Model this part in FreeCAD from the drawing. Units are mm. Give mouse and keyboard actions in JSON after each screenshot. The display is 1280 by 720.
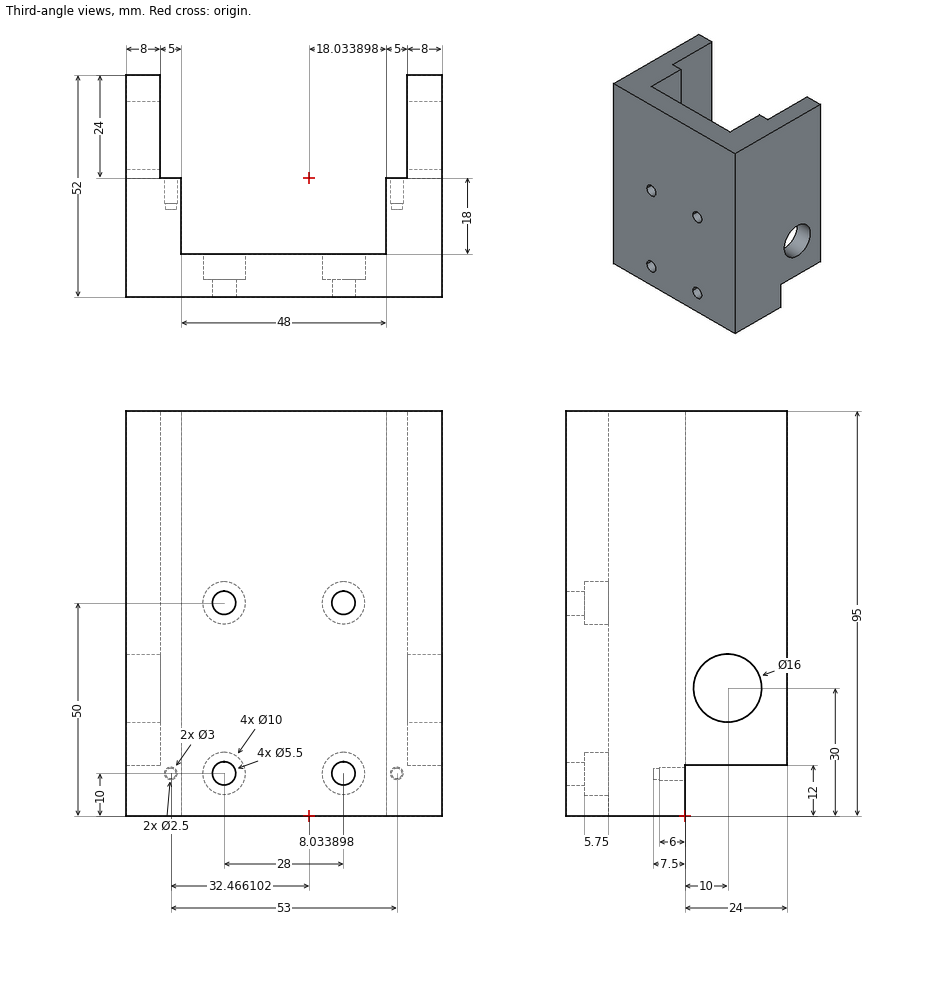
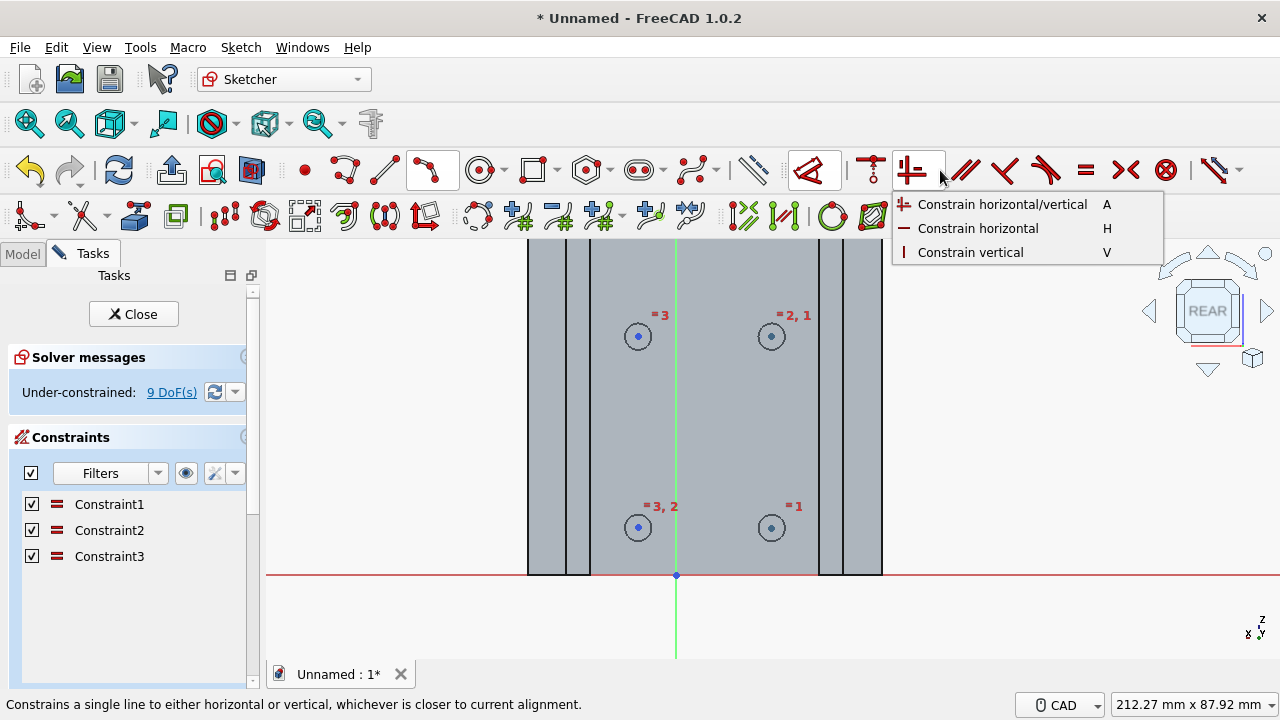
{"action": "left_click", "coordinate": [1028, 252]}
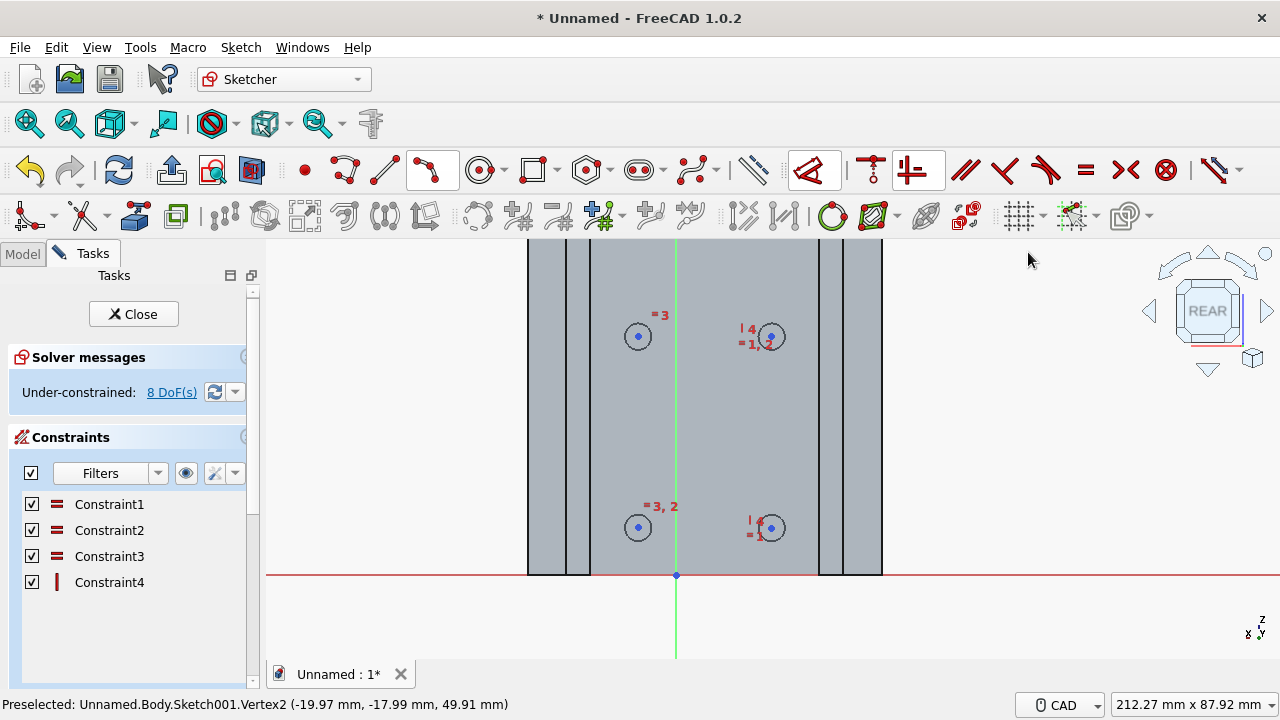
{"action": "left_click", "coordinate": [772, 528]}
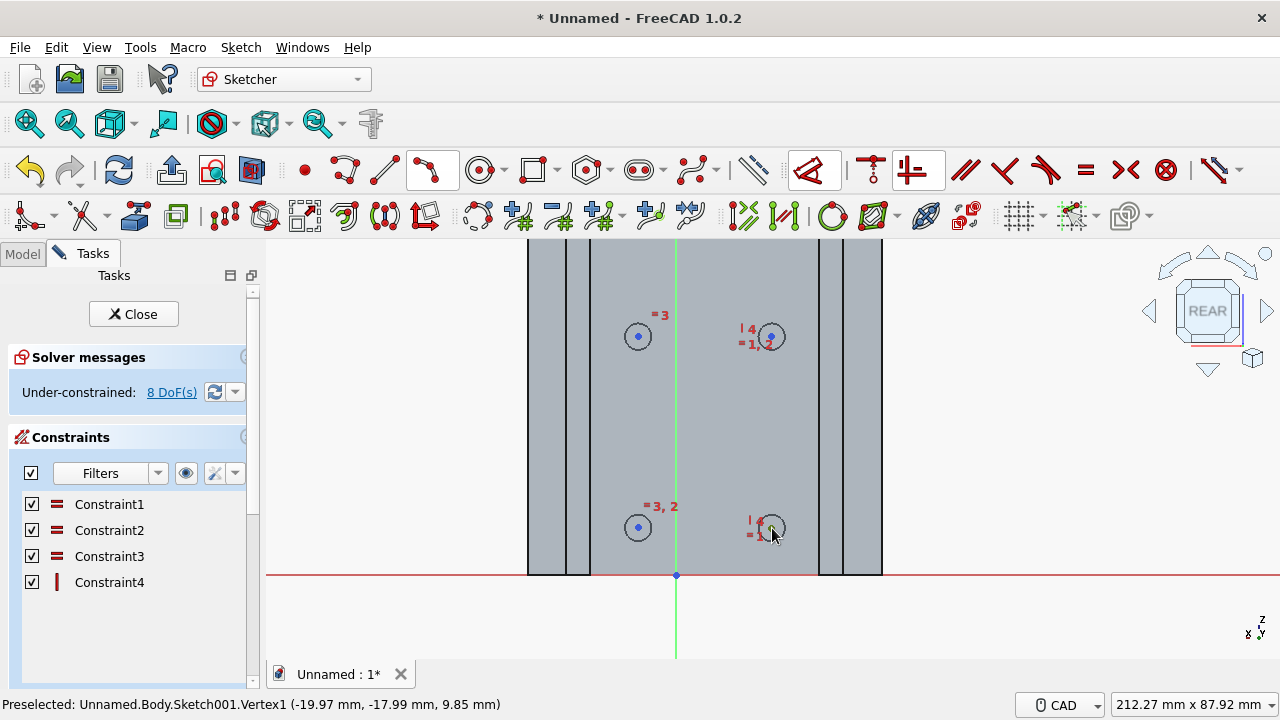
{"action": "left_click", "coordinate": [638, 528]}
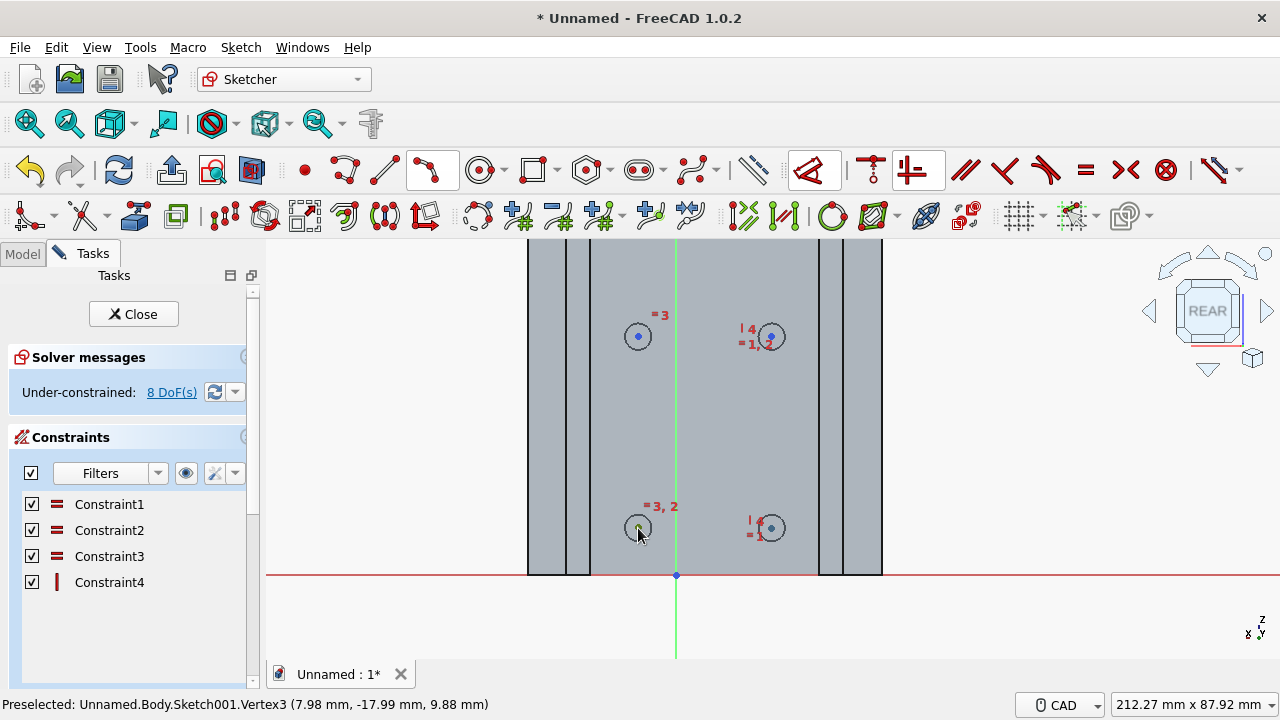
{"action": "key", "text": "h"}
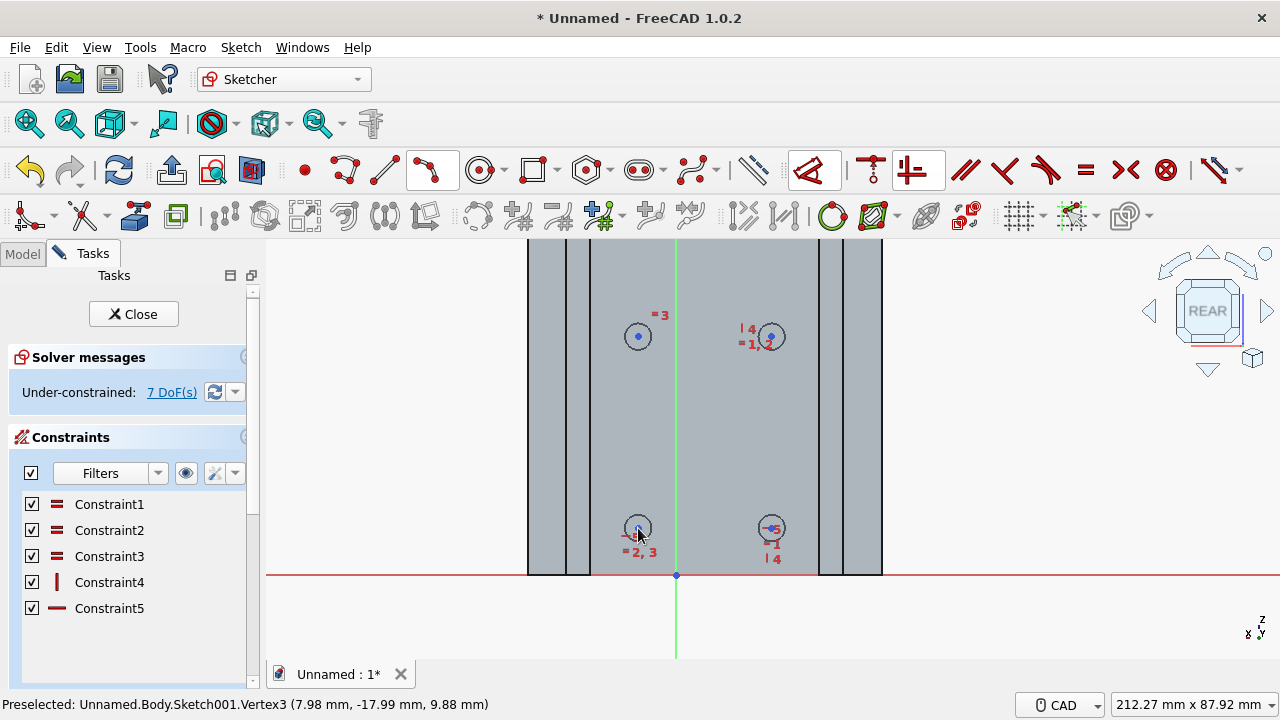
{"action": "left_click", "coordinate": [638, 528]}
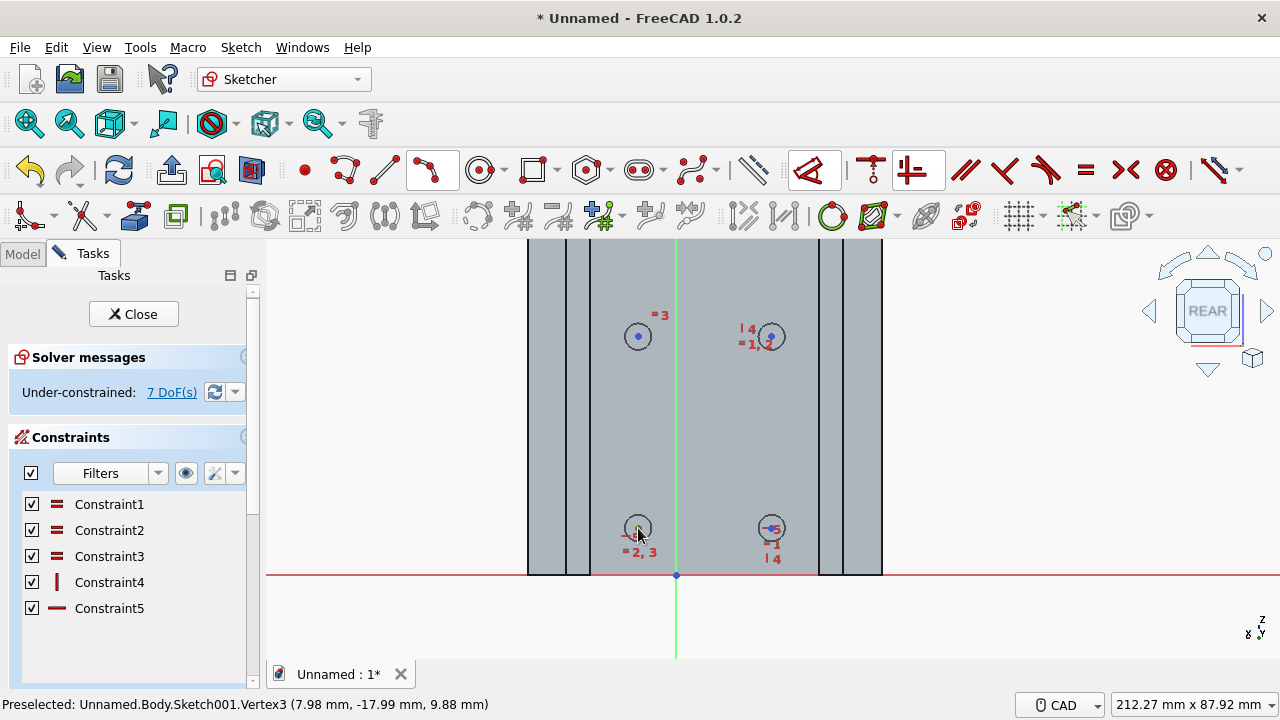
{"action": "left_click", "coordinate": [638, 337]}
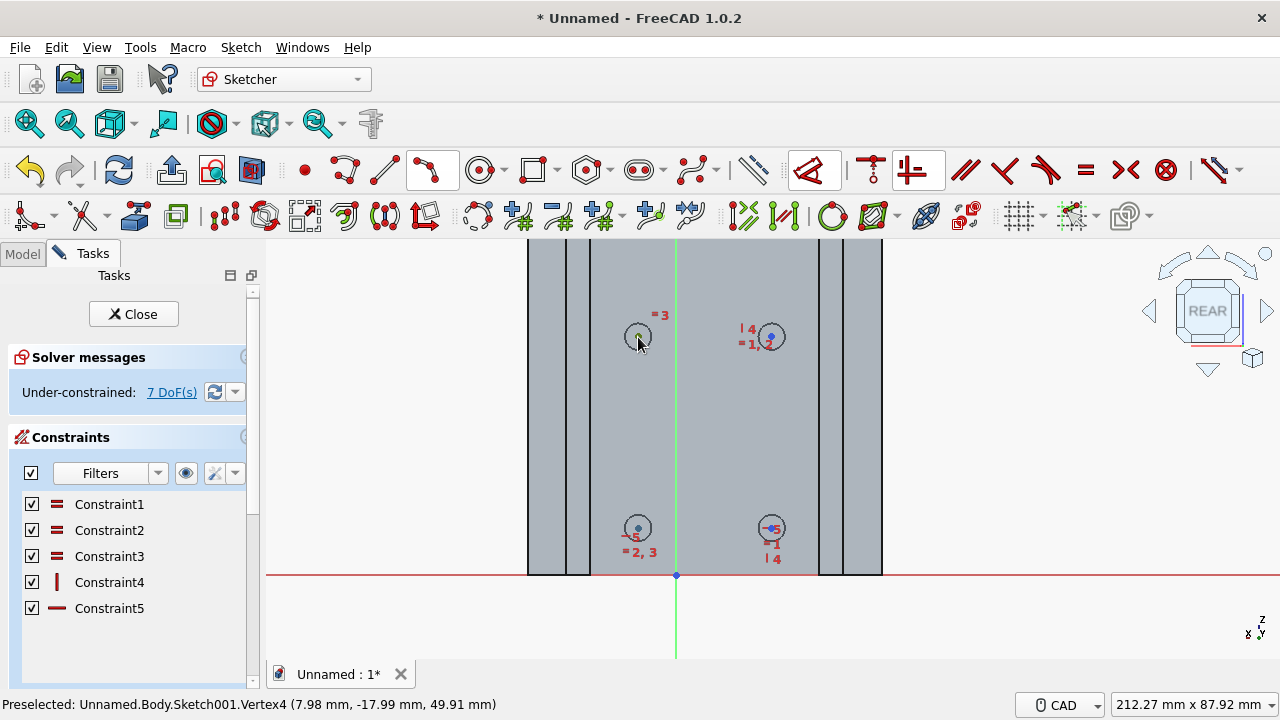
{"action": "key", "text": "v"}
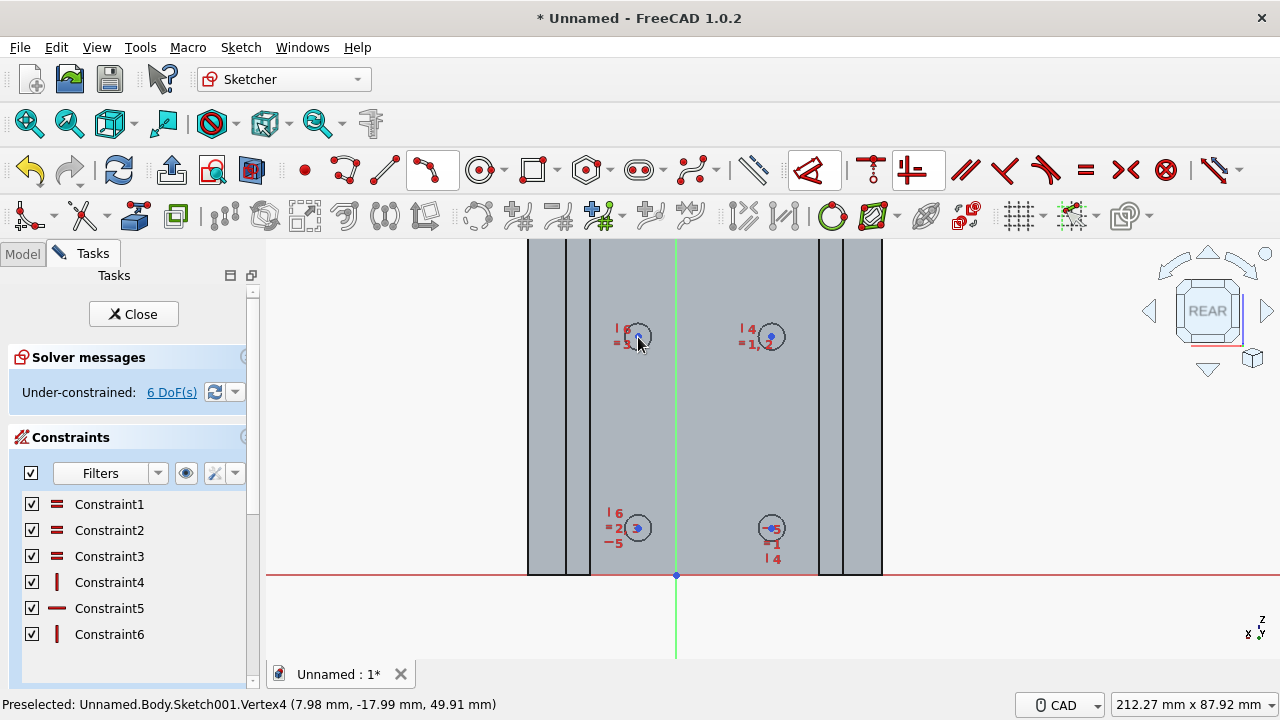
{"action": "left_click", "coordinate": [774, 339]}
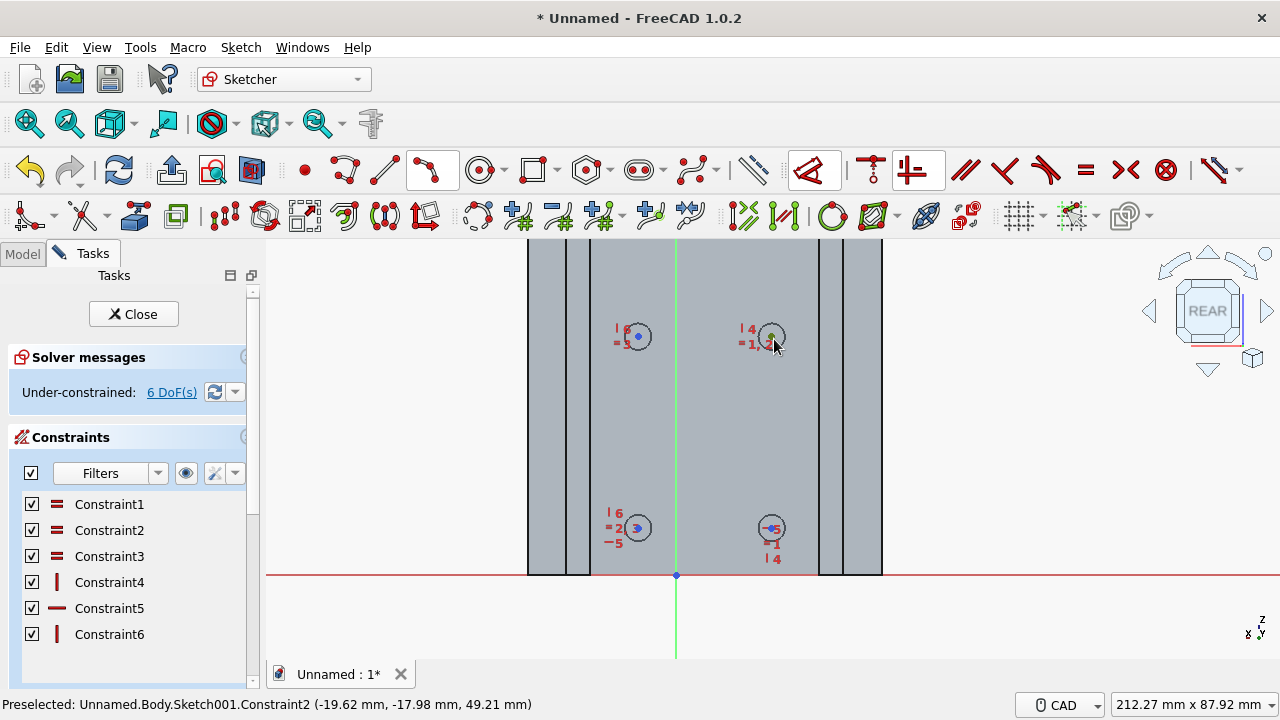
{"action": "left_click", "coordinate": [638, 337]}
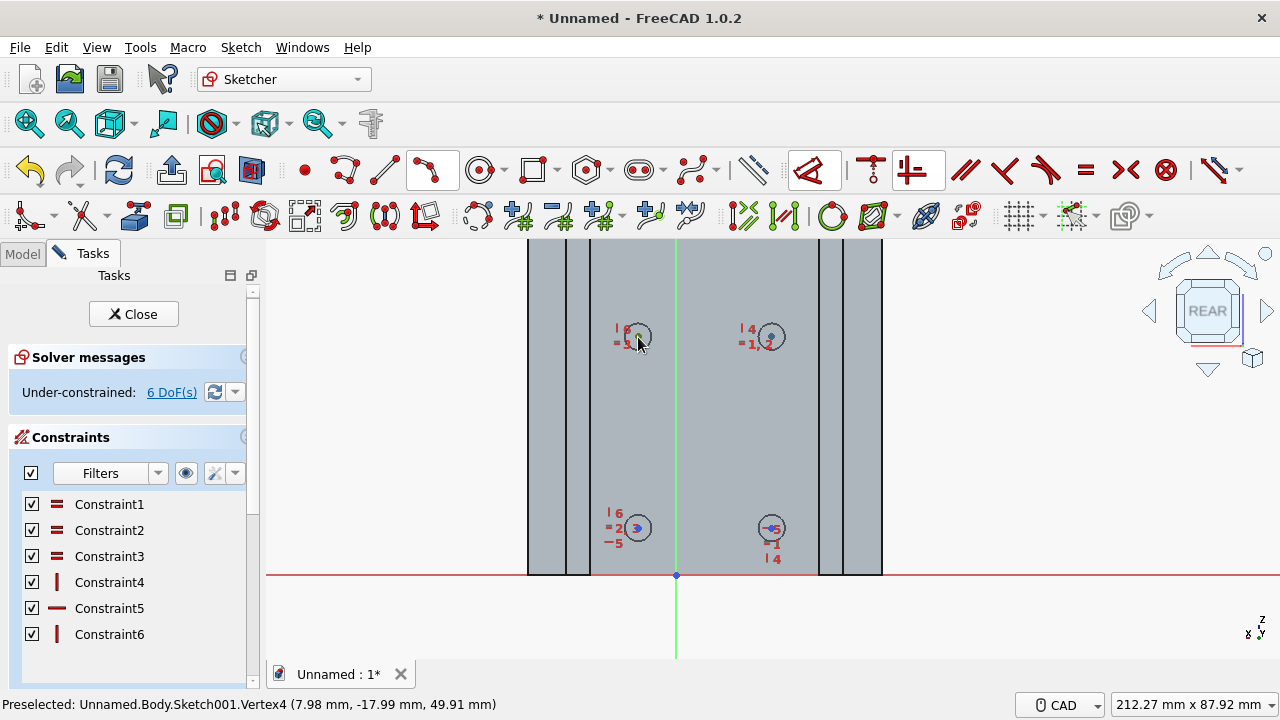
{"action": "key", "text": "h"}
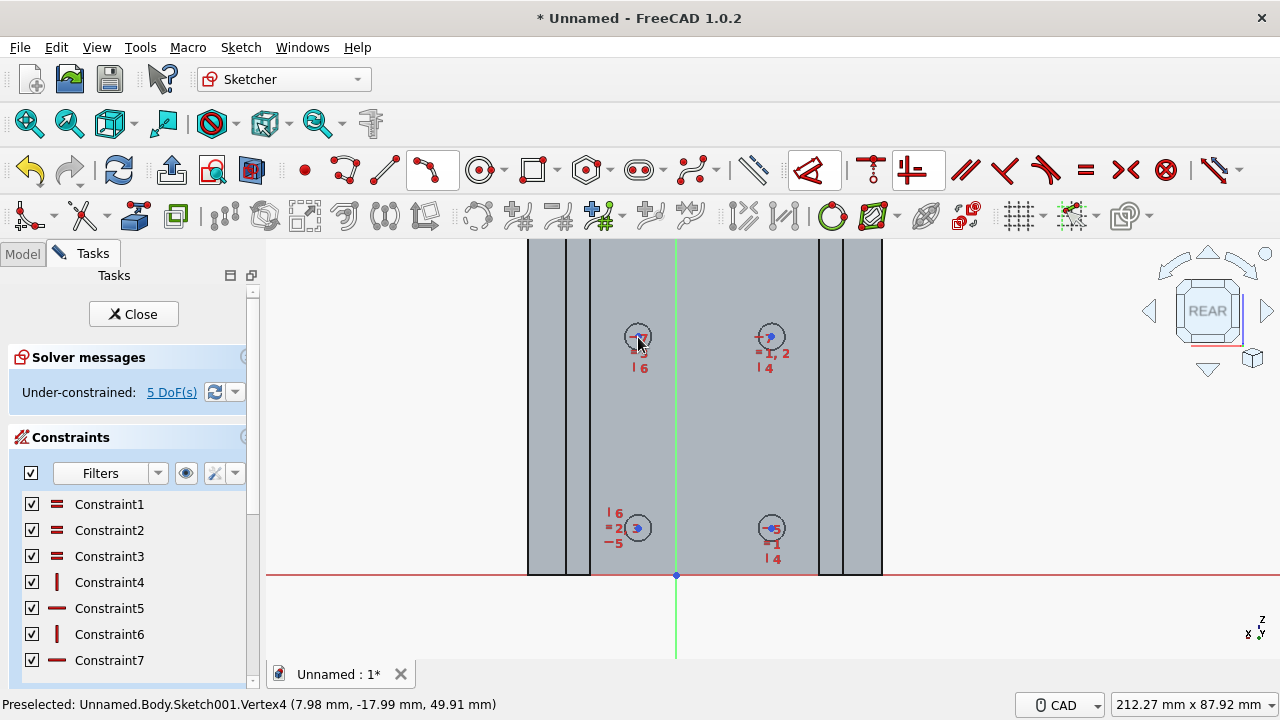
{"action": "scroll", "coordinate": [781, 519], "scroll_direction": "up", "scroll_amount": 3}